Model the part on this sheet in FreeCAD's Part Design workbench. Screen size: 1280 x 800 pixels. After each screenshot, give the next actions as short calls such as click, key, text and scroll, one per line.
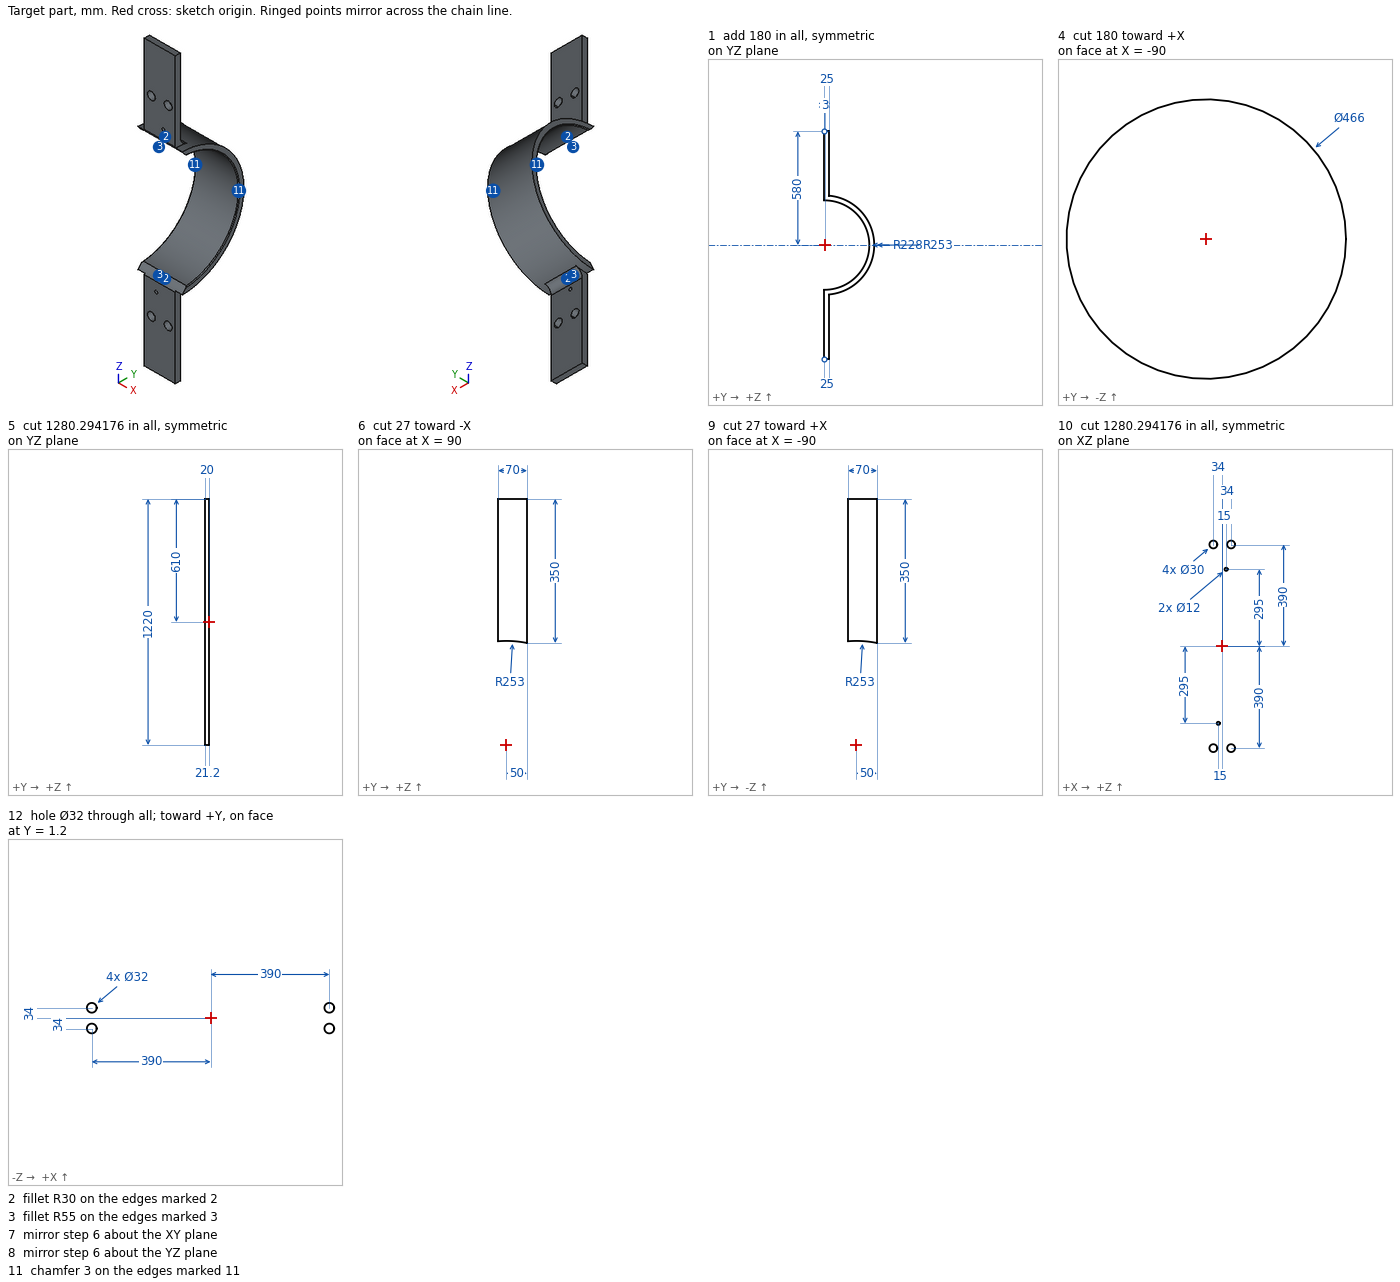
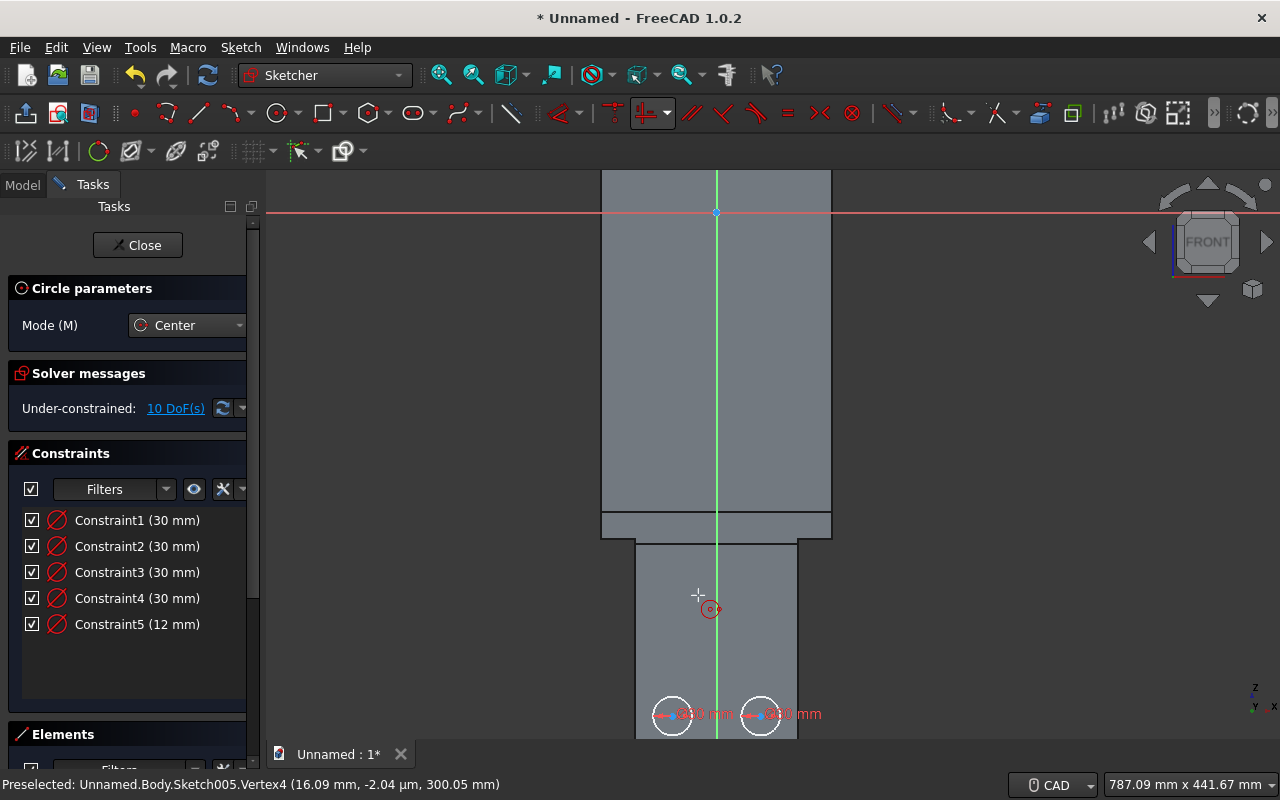
click(697, 593)
move(692, 588)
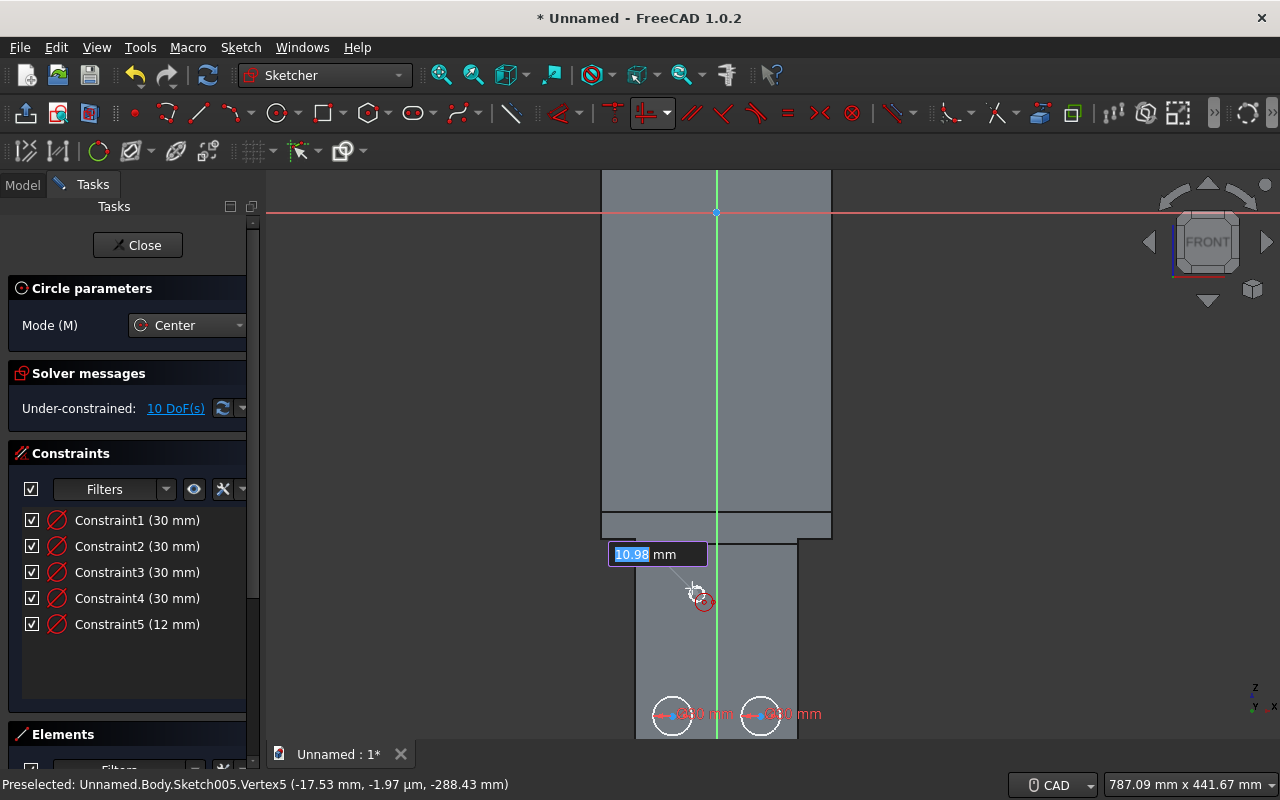
text(12)
key(Return)
key(Escape)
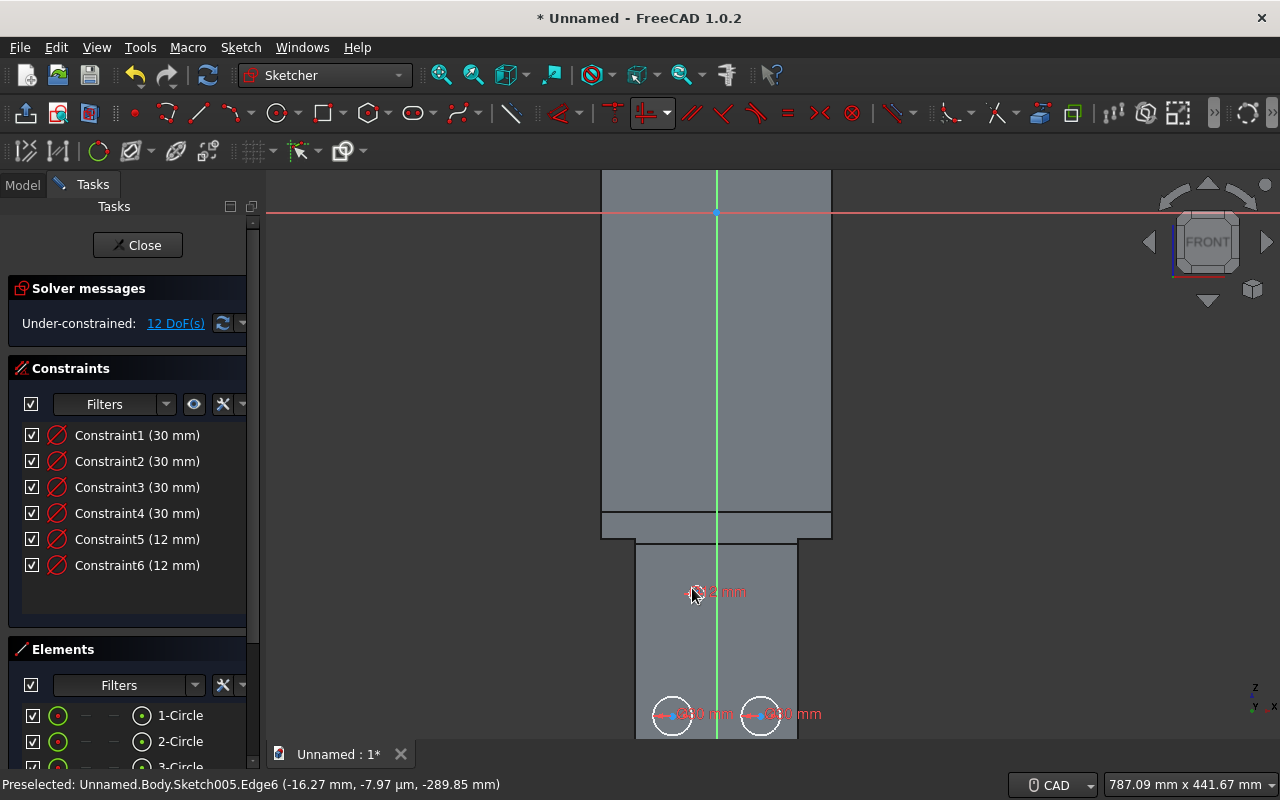
scroll(698, 595, down, 5)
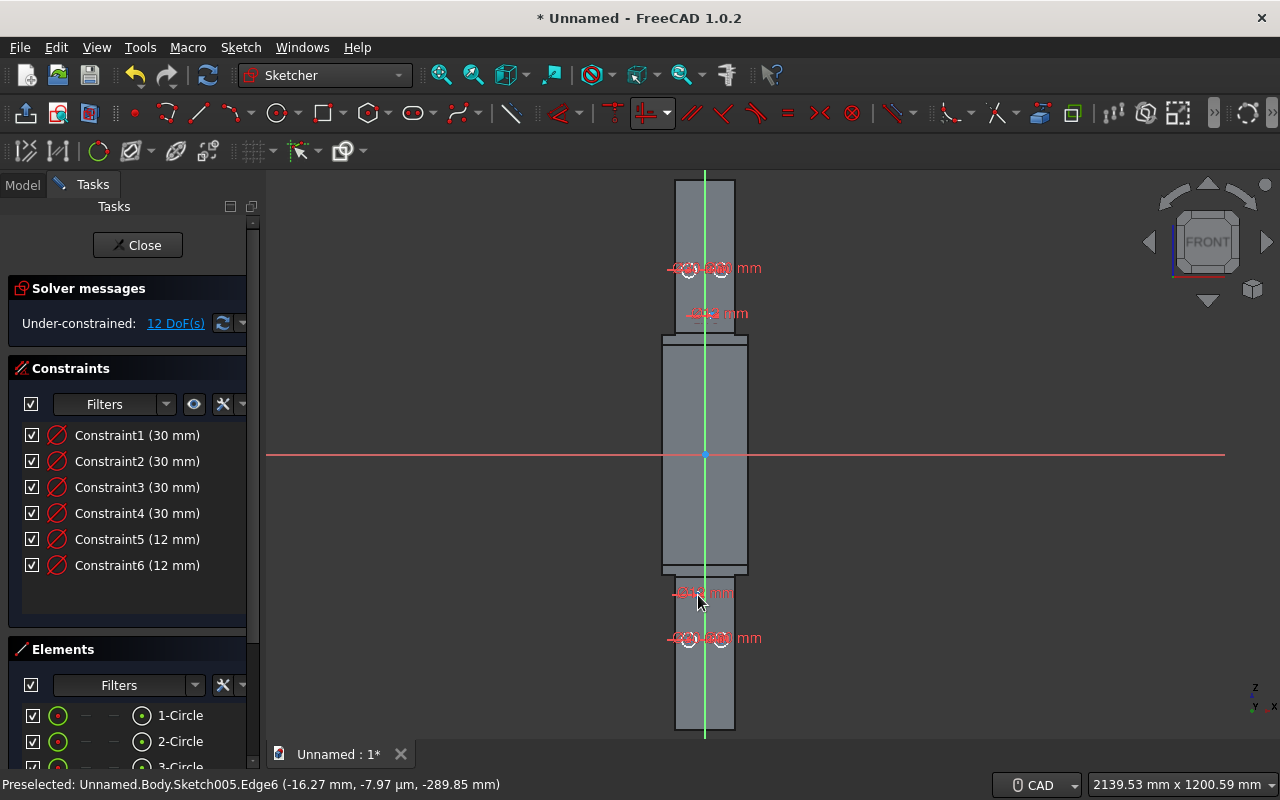
click(721, 270)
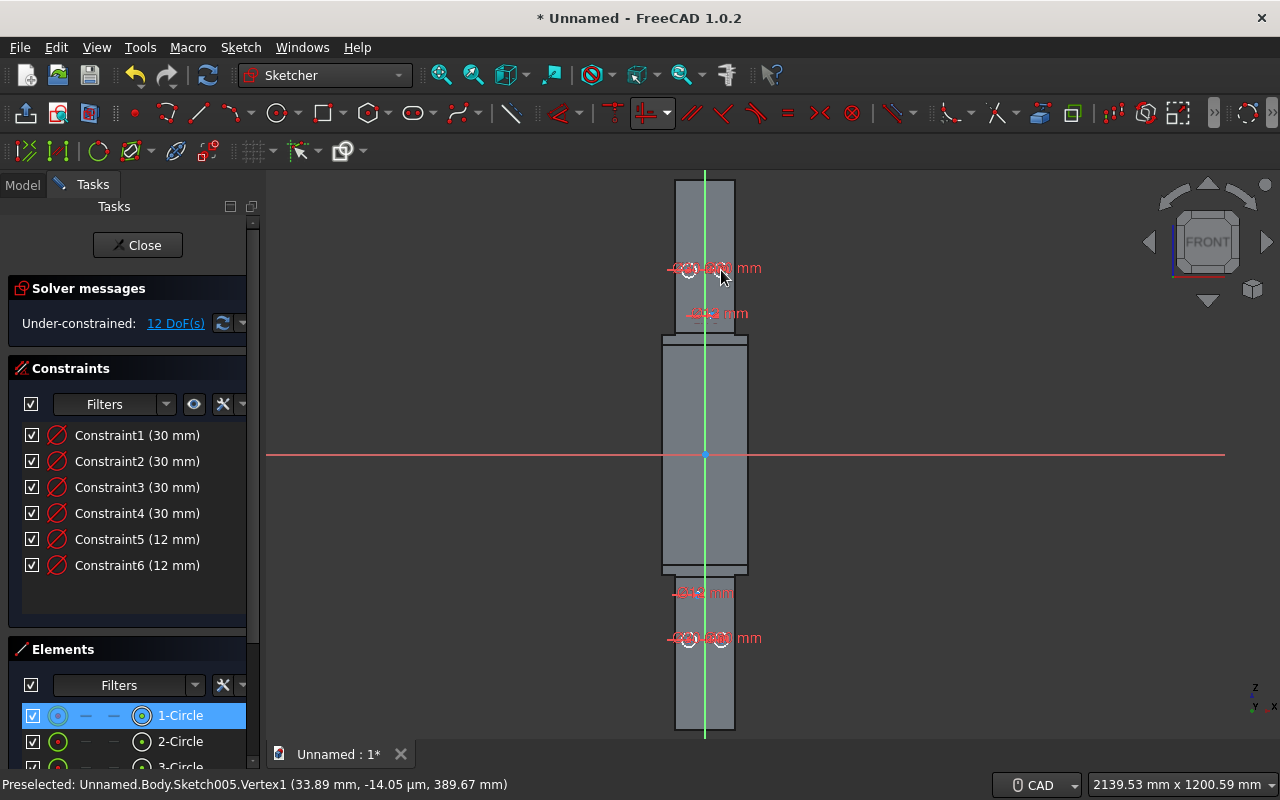
click(721, 640)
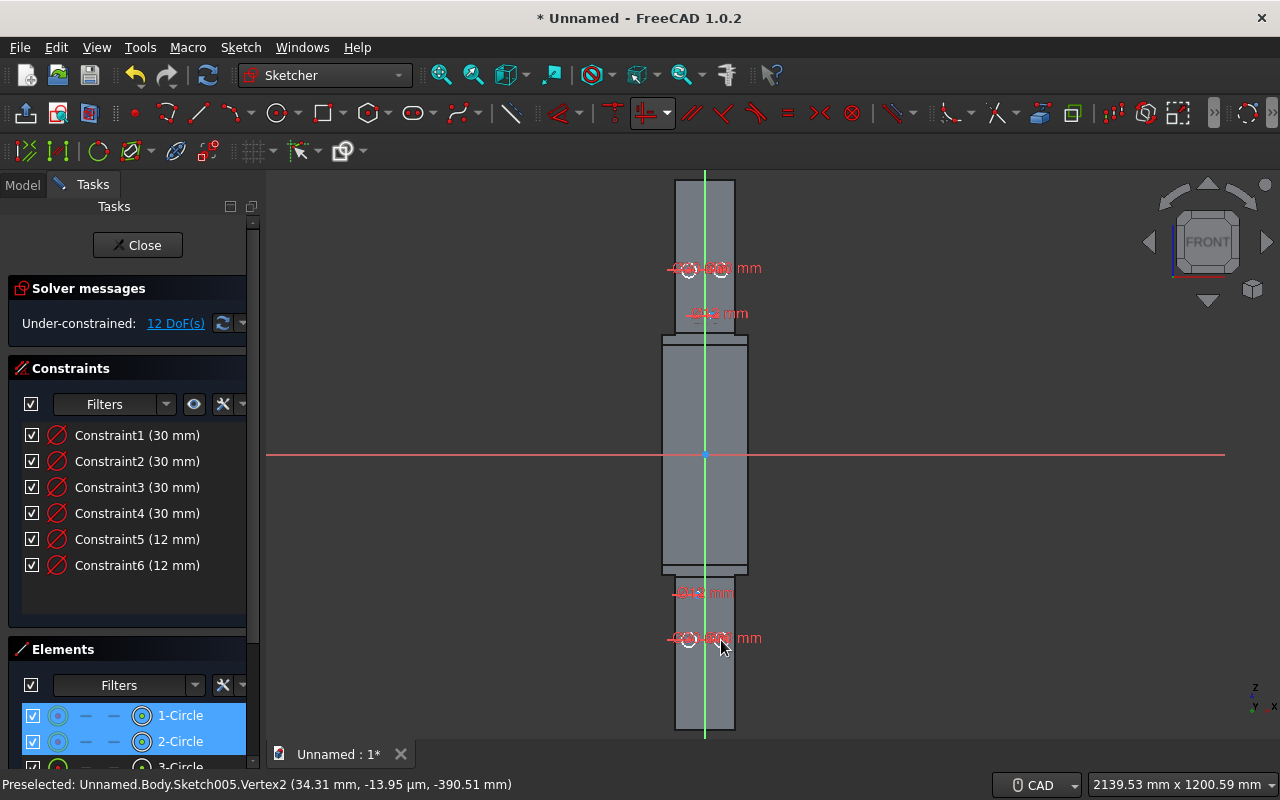
click(670, 114)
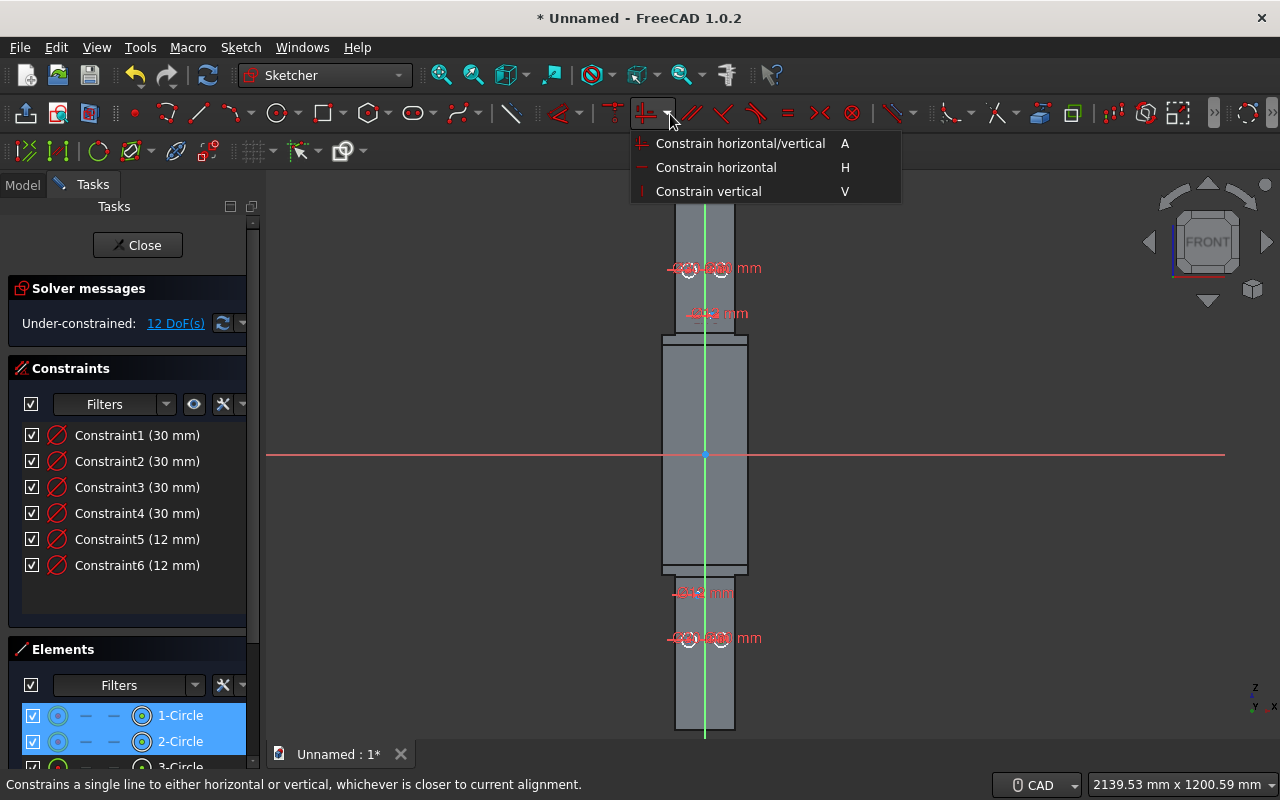
click(766, 191)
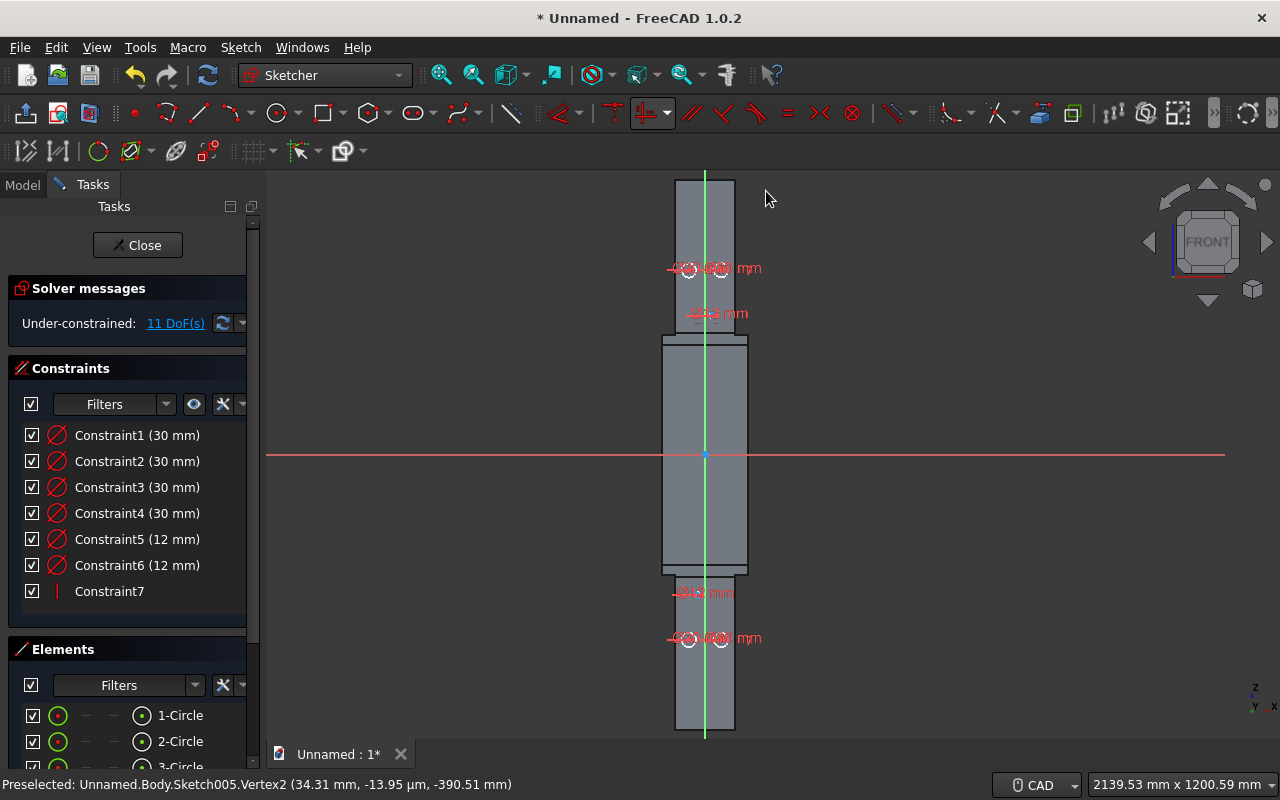
click(721, 270)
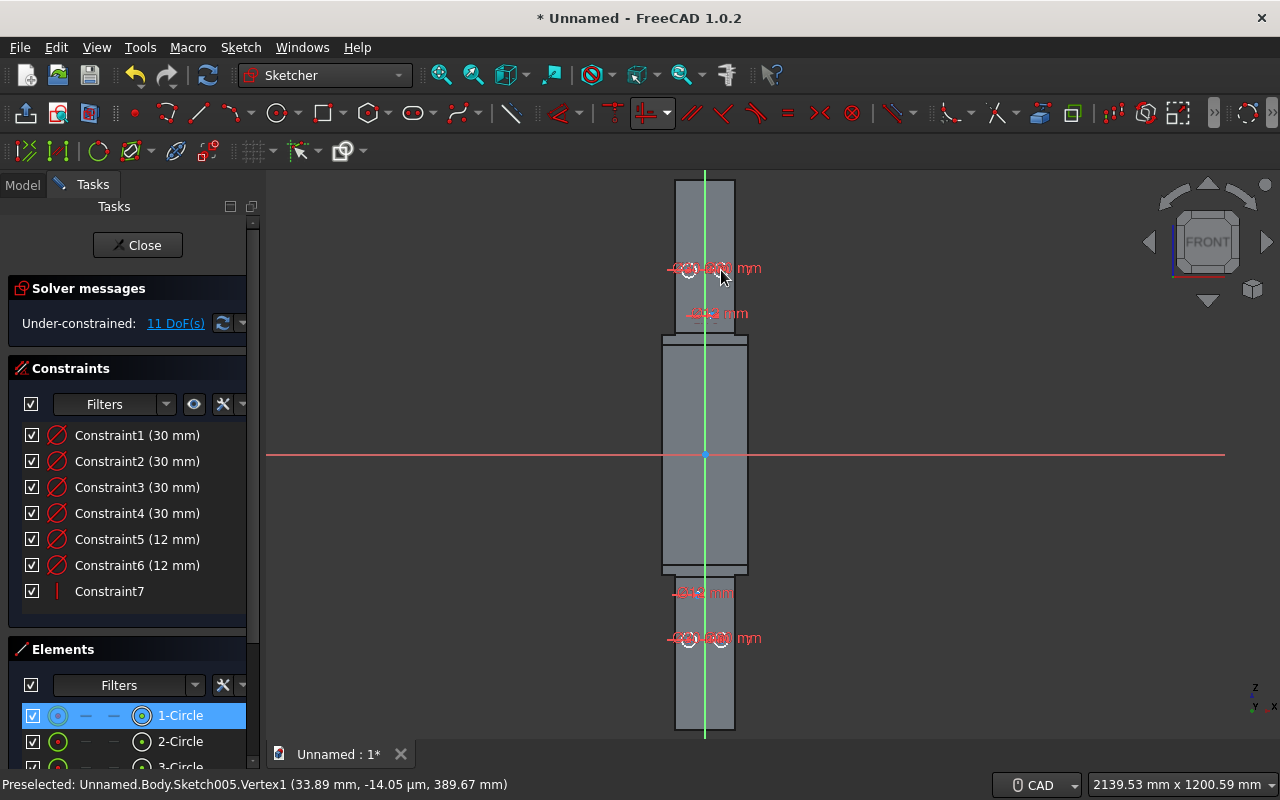
click(689, 270)